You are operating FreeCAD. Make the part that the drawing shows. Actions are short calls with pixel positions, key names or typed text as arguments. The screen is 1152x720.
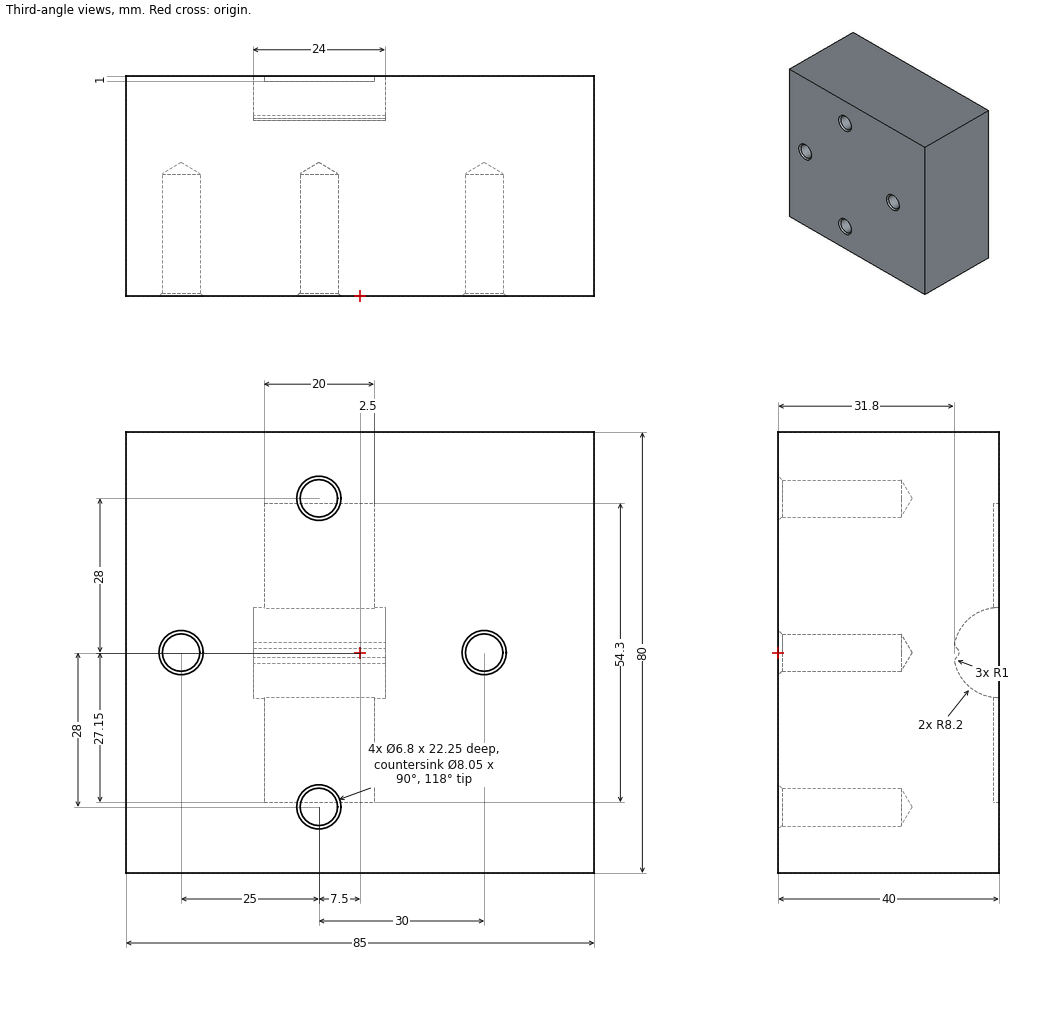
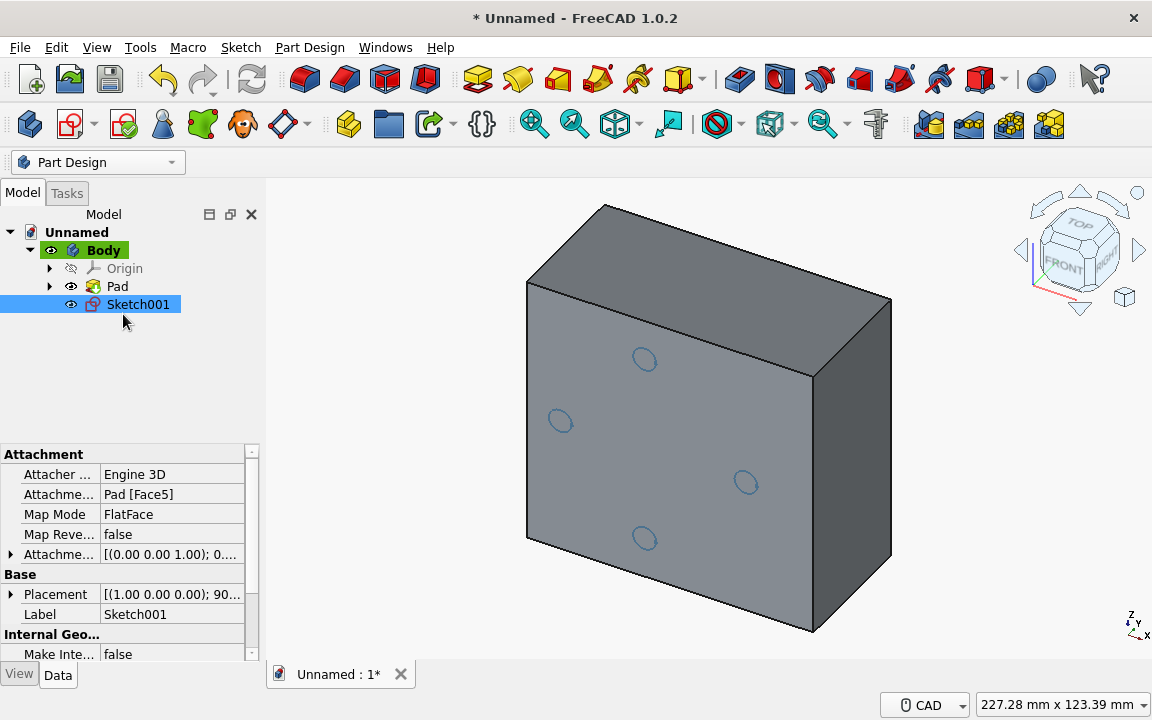
click(780, 80)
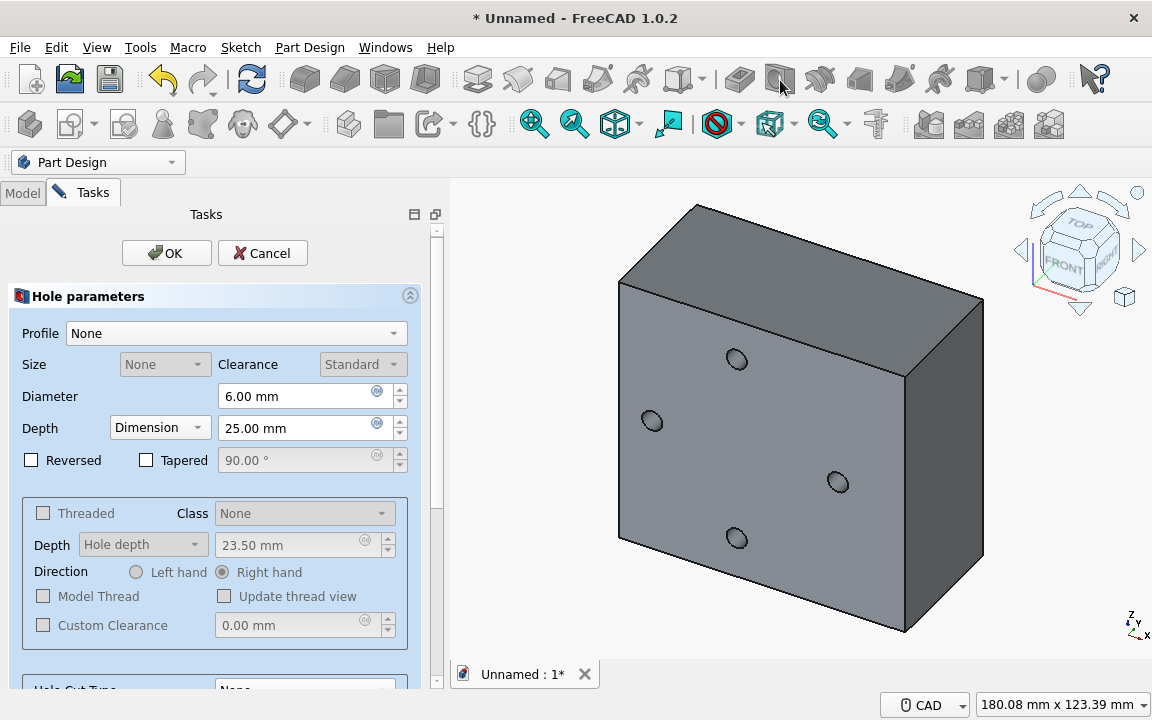
triple_click(305, 396)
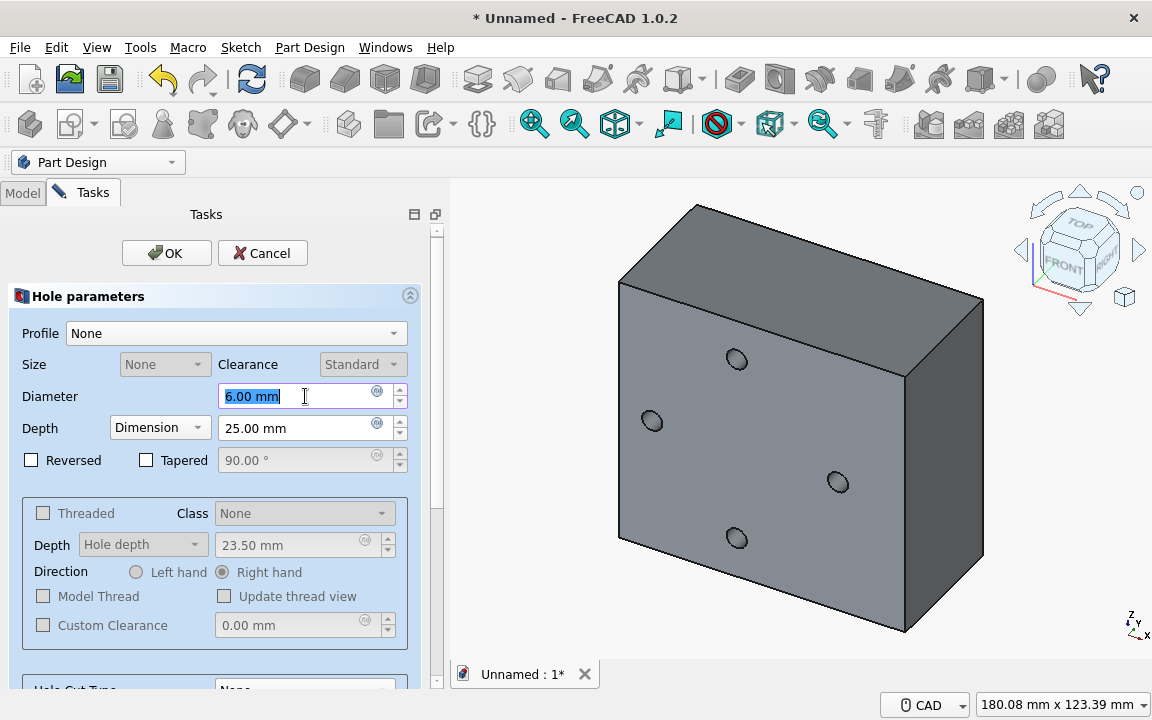
text(6.8)
key(Tab)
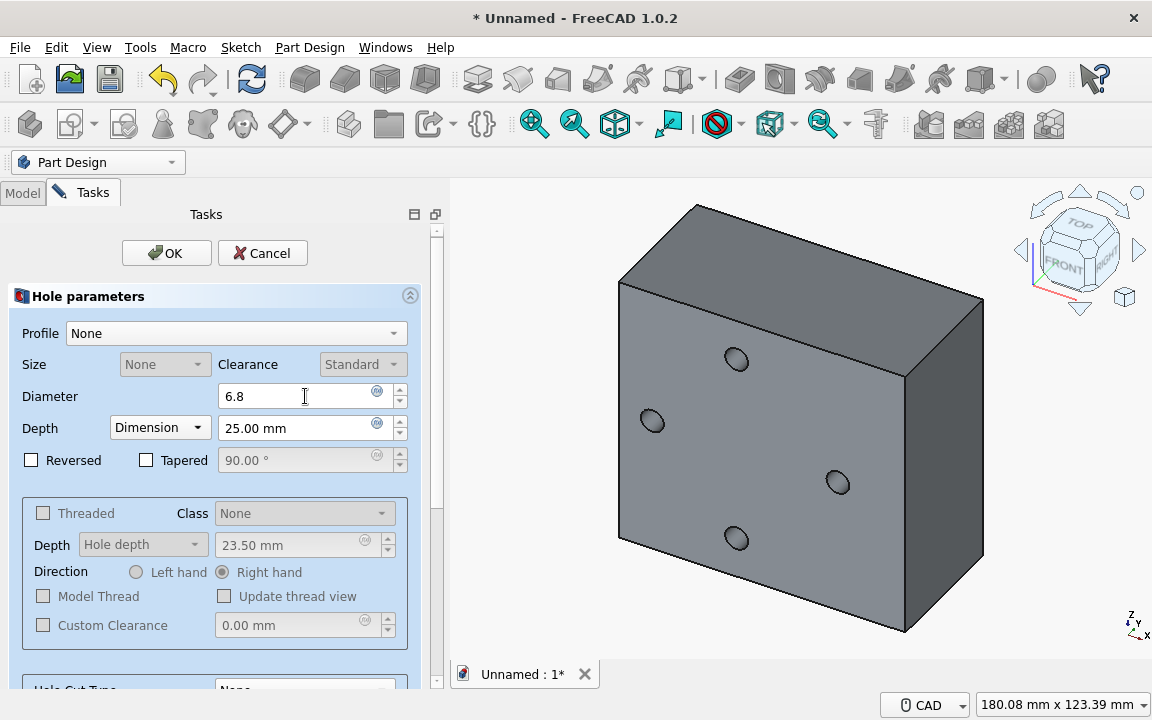
triple_click(305, 428)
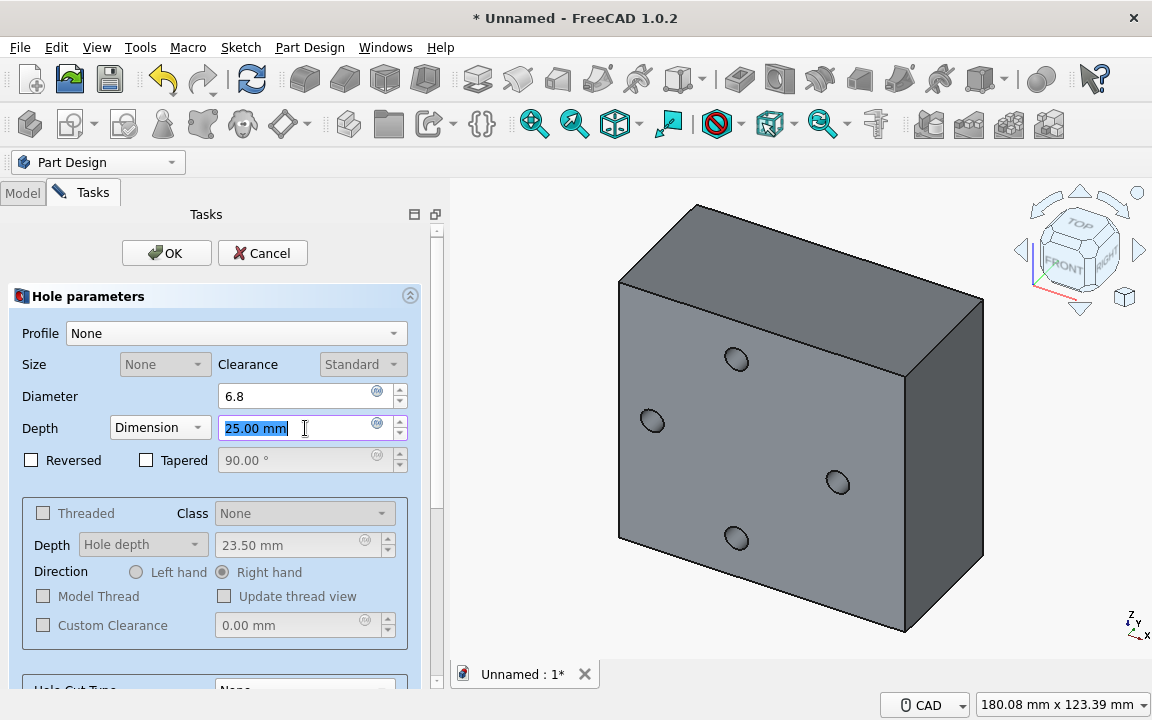
text(22.25)
key(Tab)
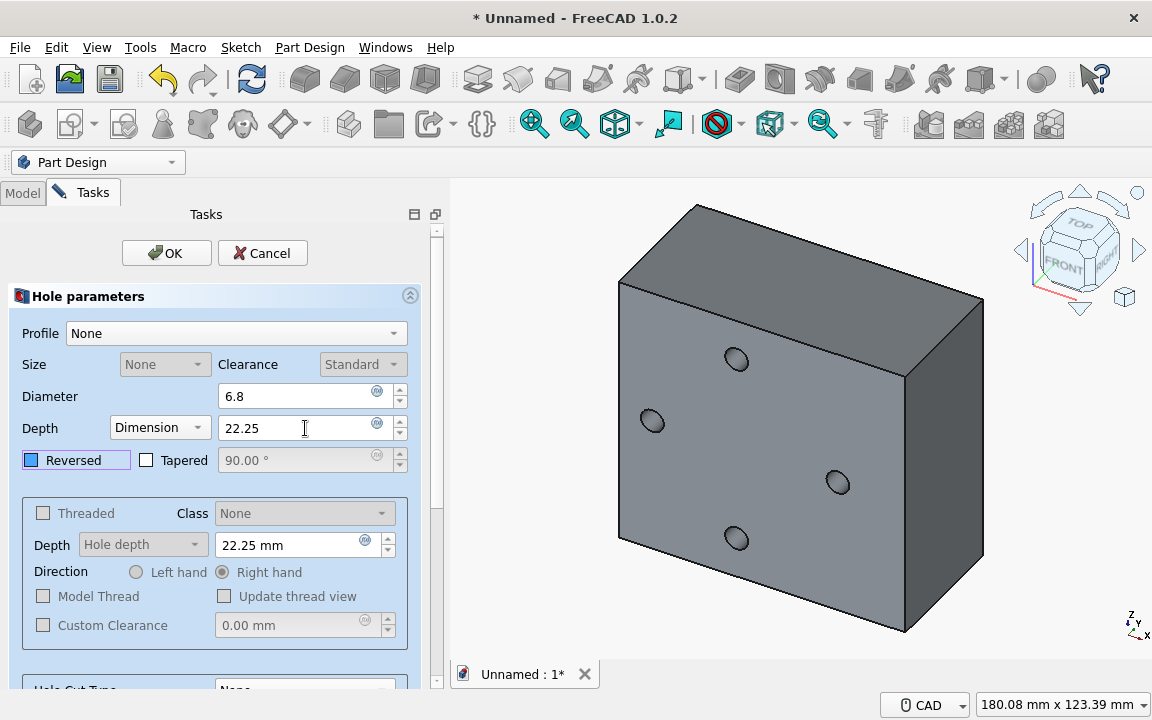
scroll(437, 456, down, 2)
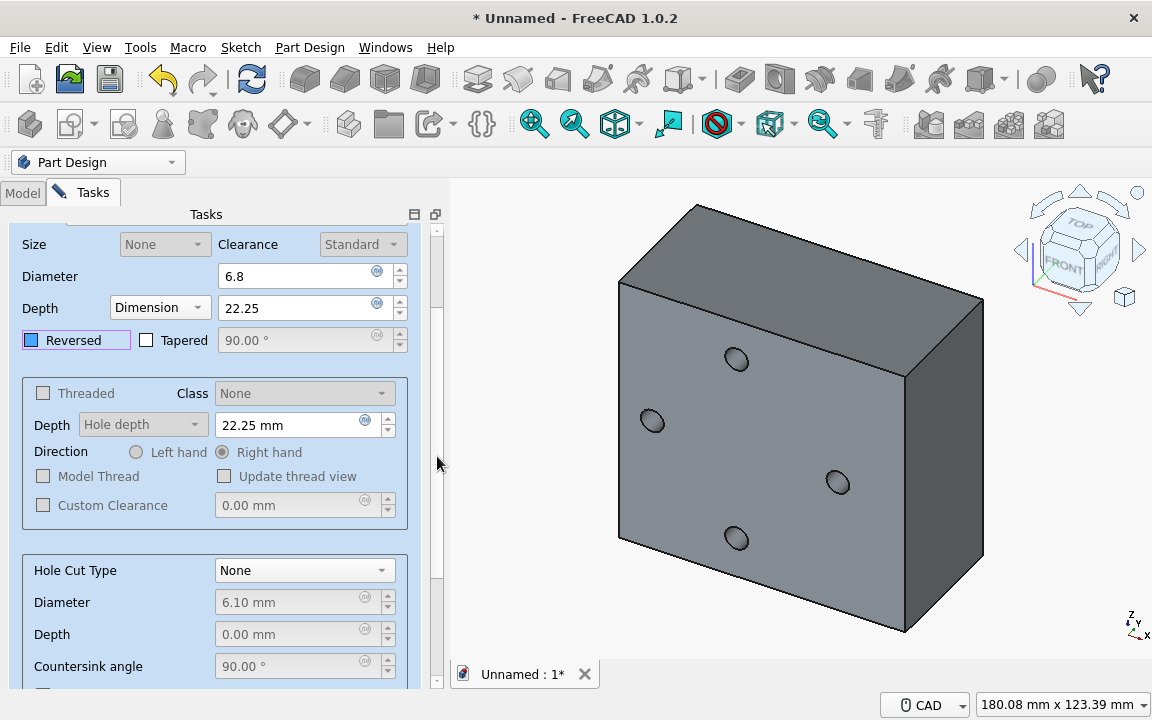
click(306, 570)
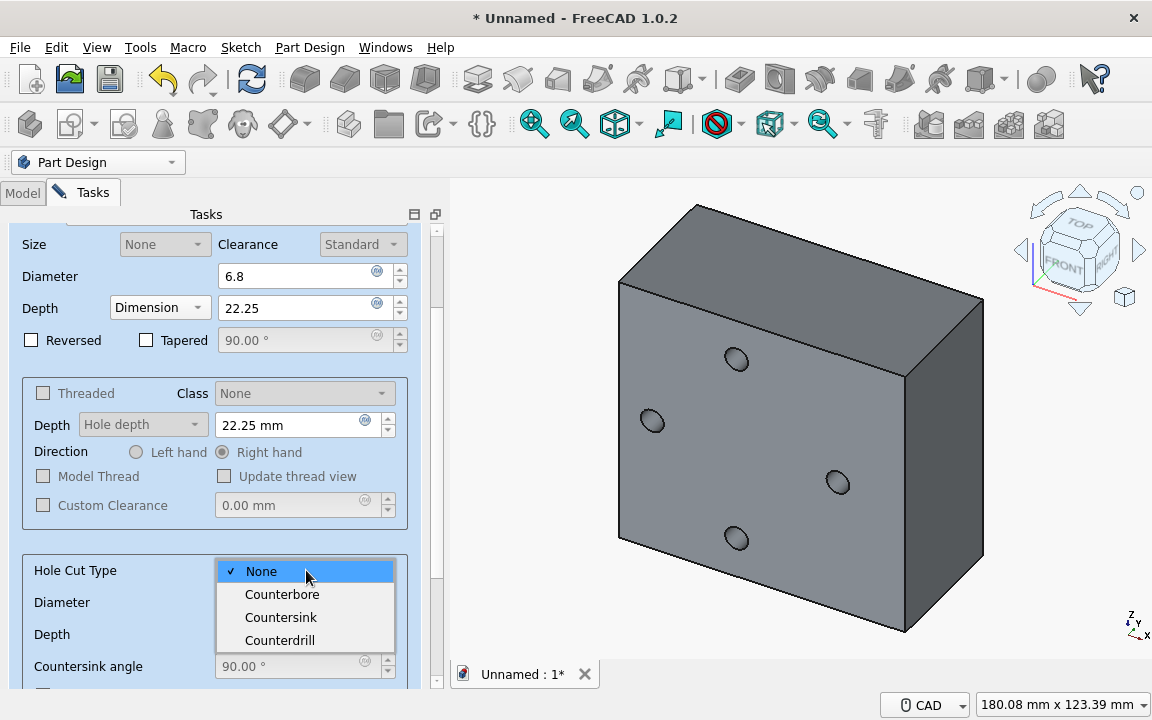
click(304, 618)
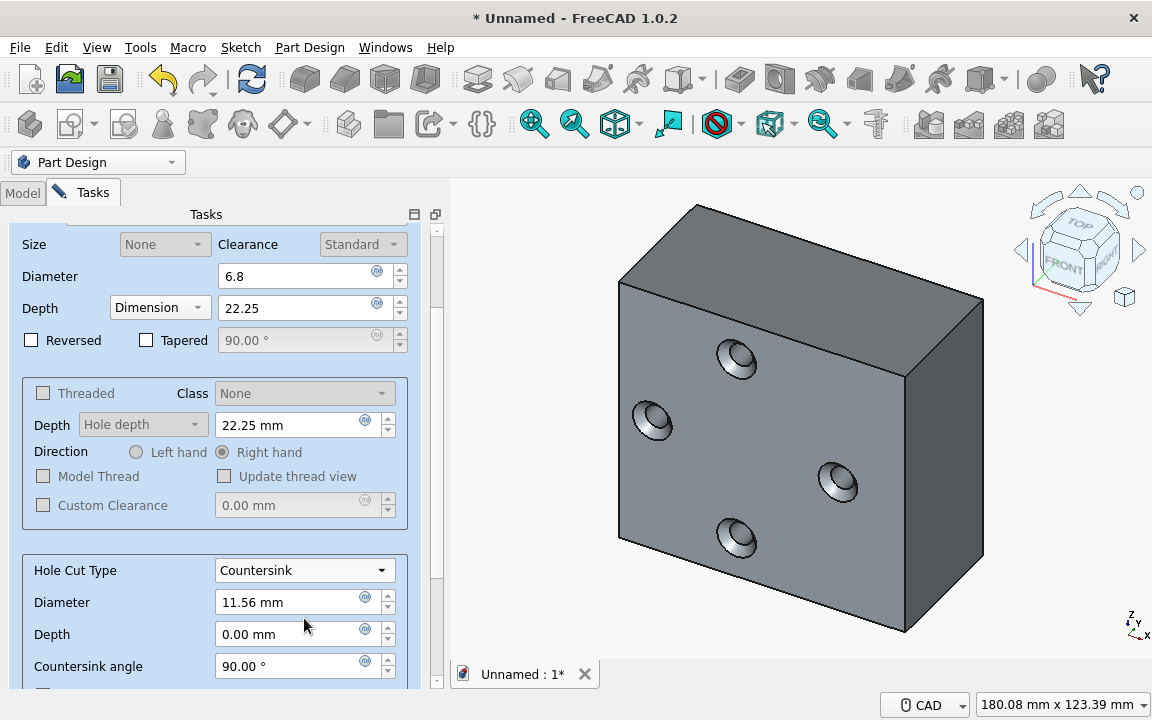
triple_click(298, 602)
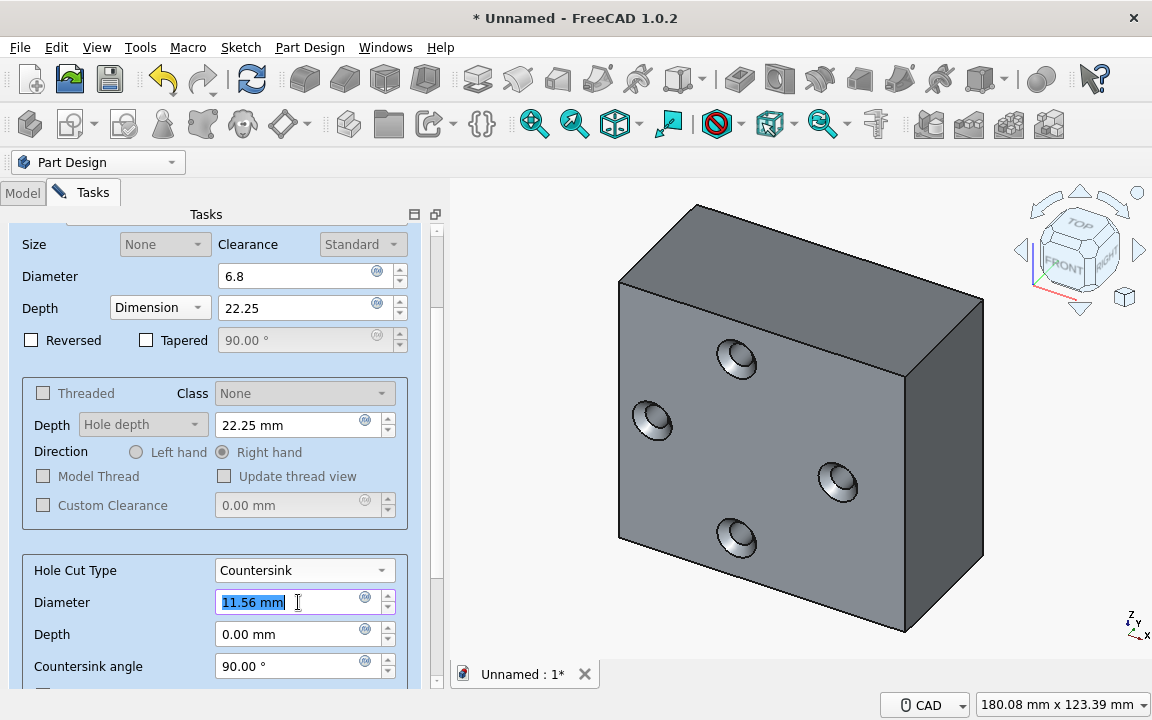
text(8.05)
key(Tab)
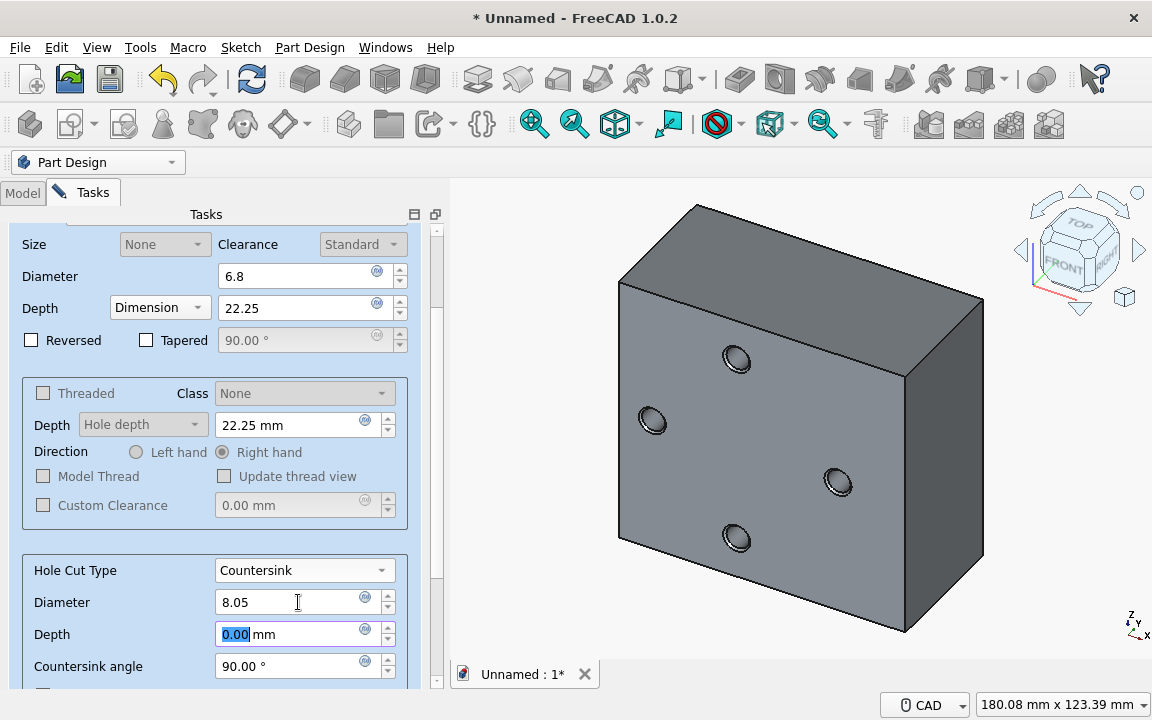
scroll(437, 456, up, 3)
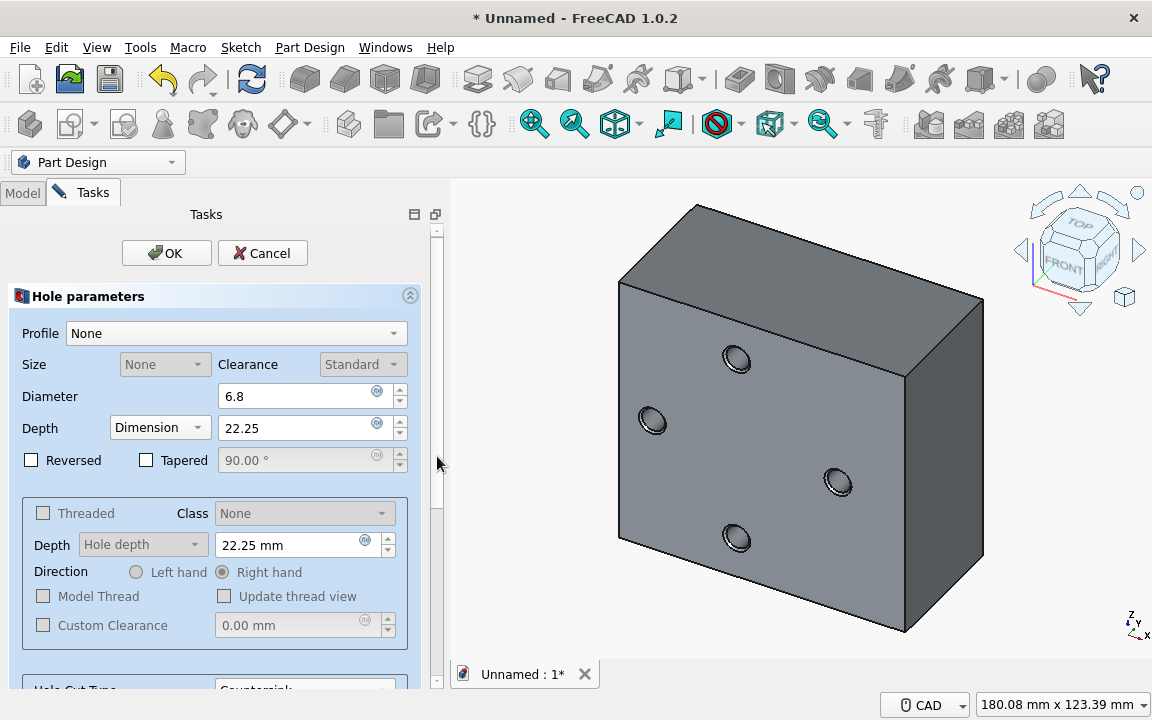
click(167, 253)